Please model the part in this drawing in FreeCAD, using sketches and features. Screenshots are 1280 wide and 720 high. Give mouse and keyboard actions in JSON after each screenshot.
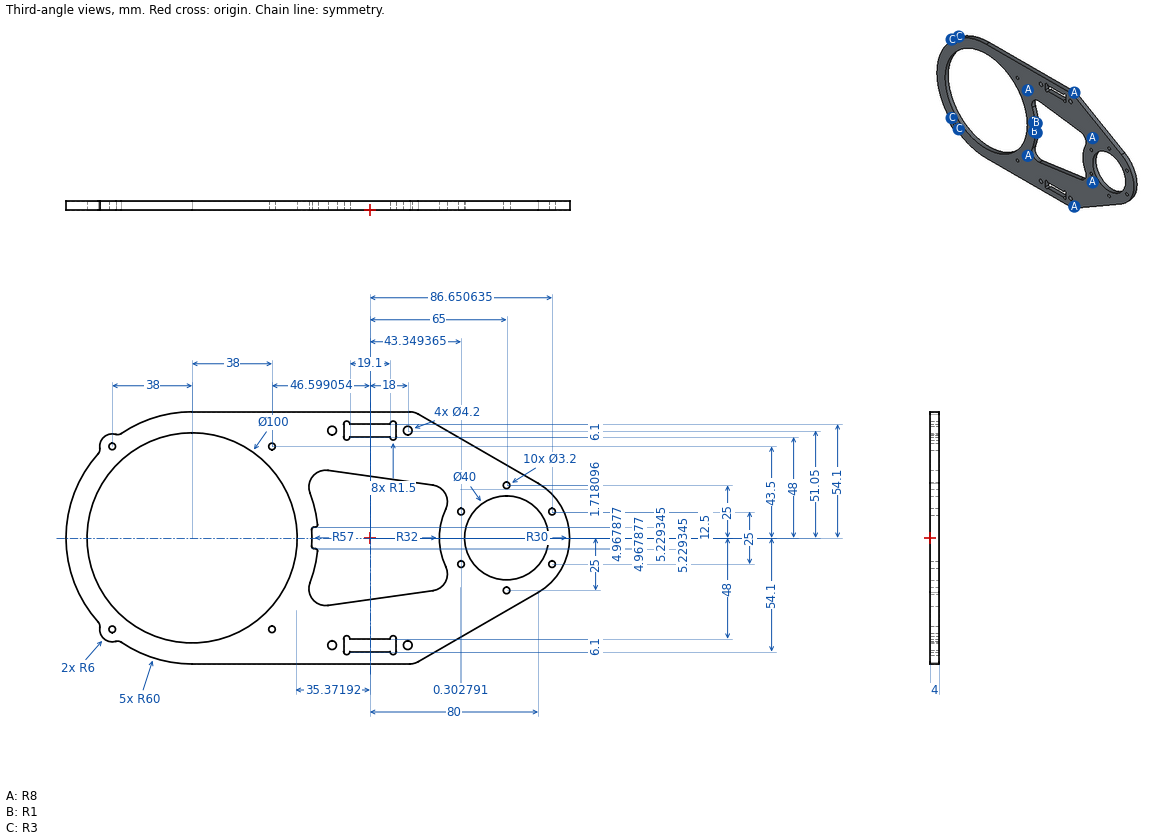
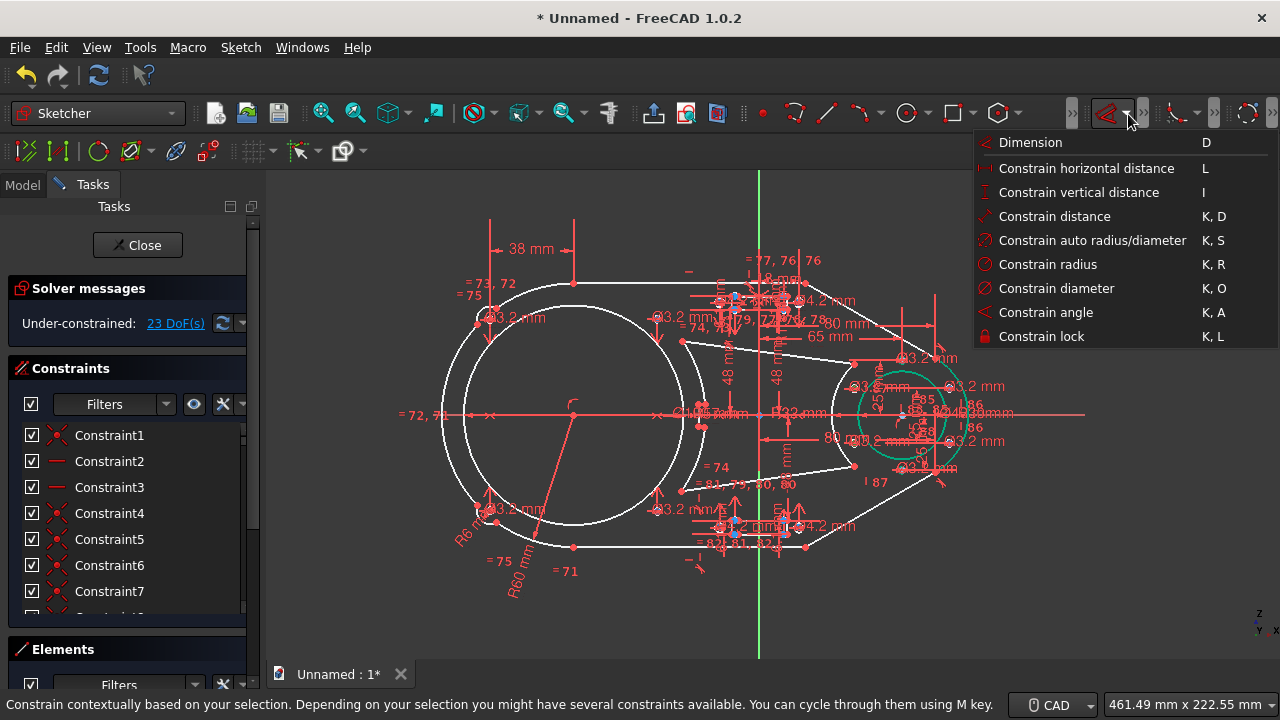
{"action": "left_click", "coordinate": [1126, 192]}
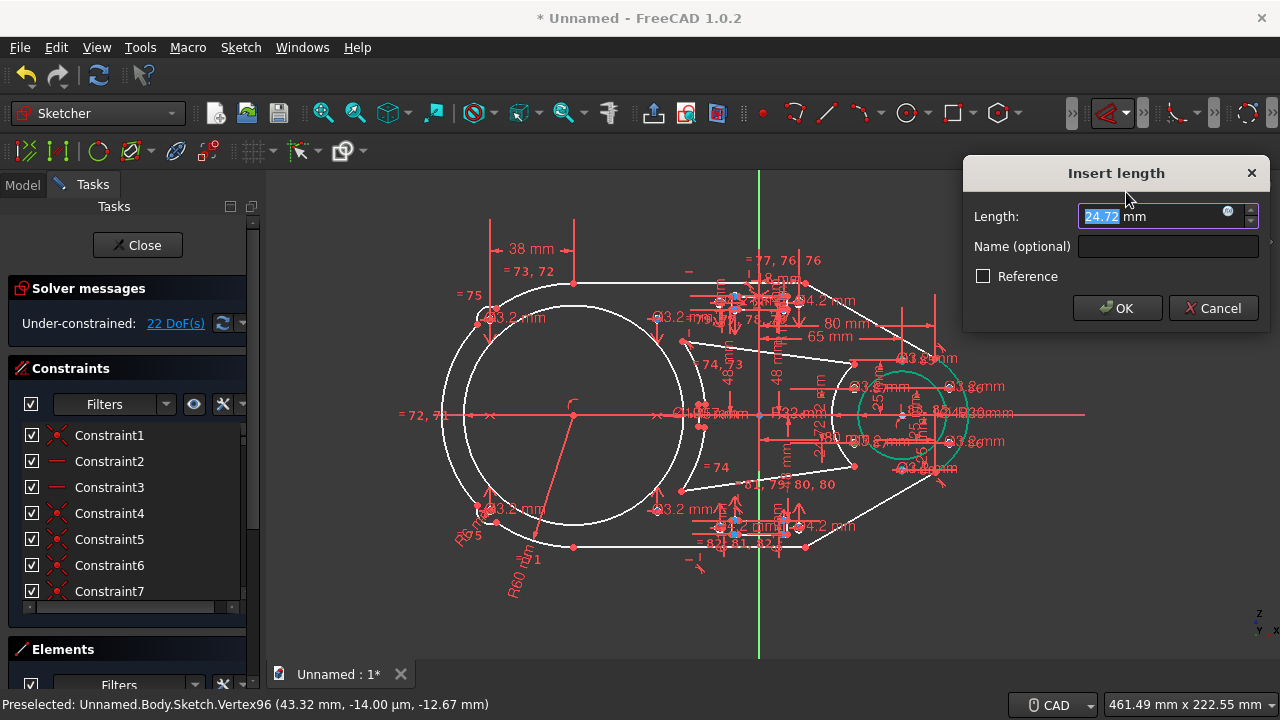
{"action": "type", "text": "25"}
{"action": "key", "text": "Return"}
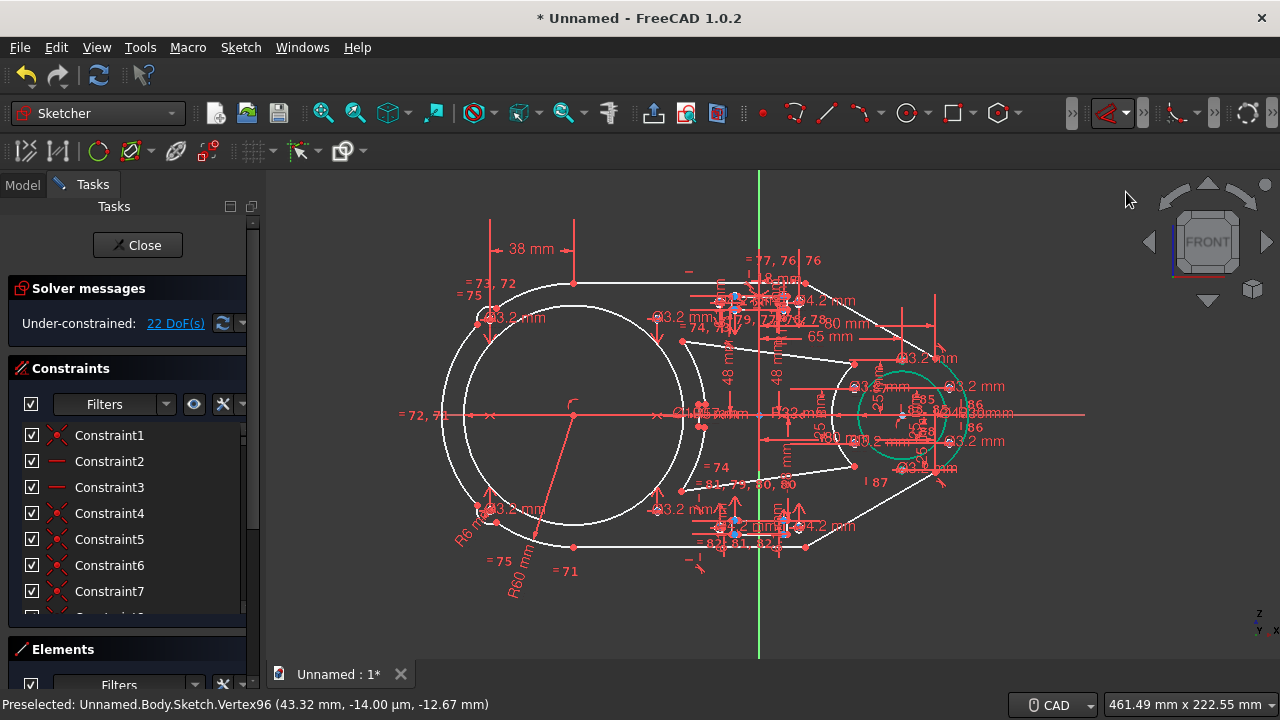
{"action": "left_click", "coordinate": [490, 320]}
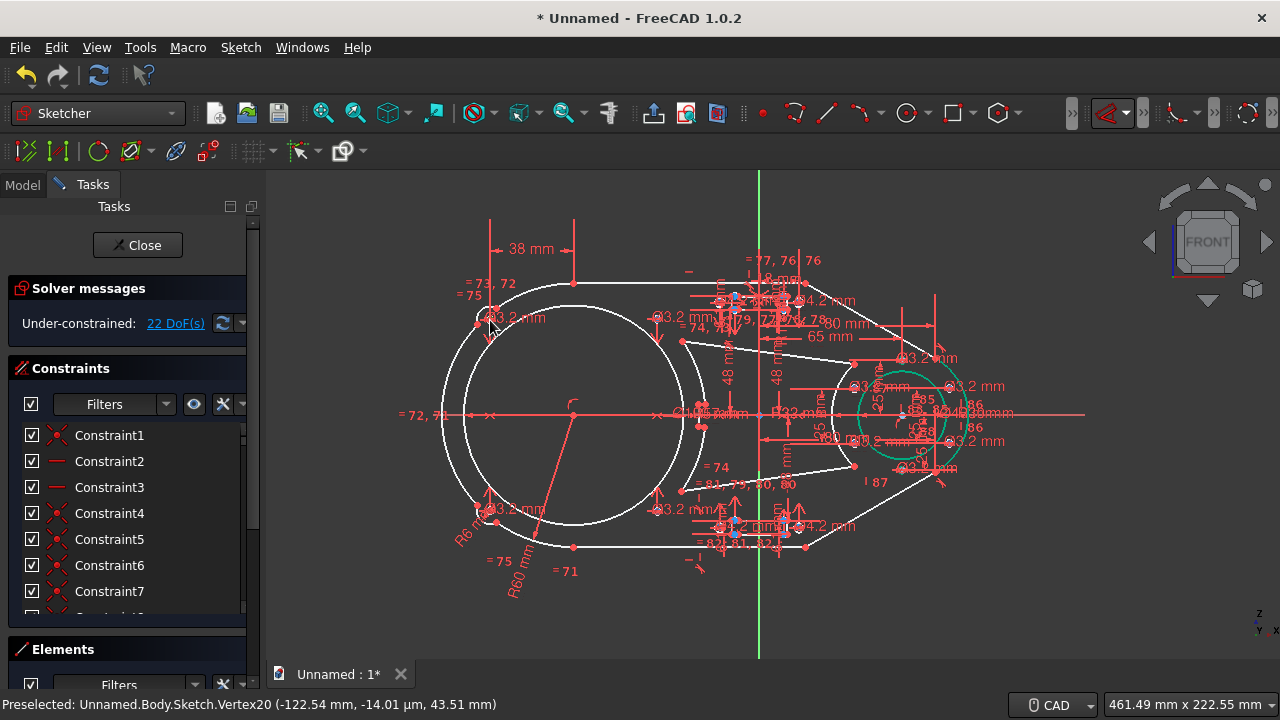
{"action": "left_click", "coordinate": [574, 415]}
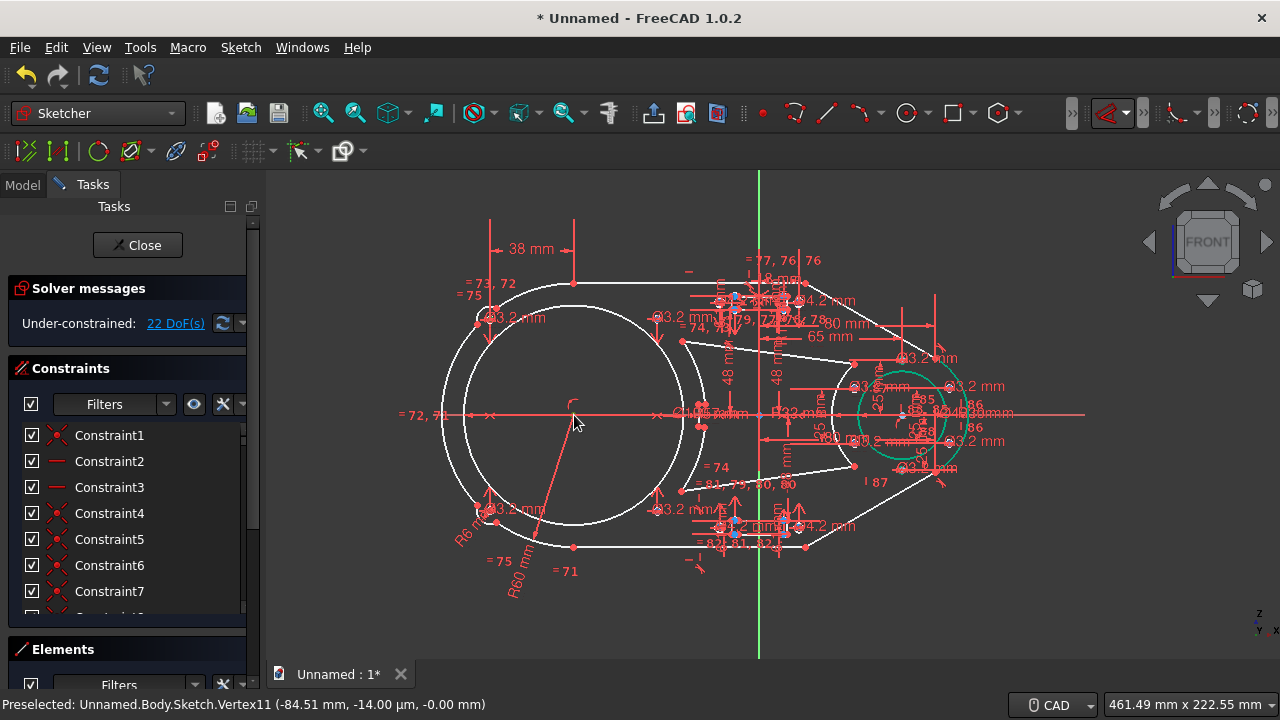
{"action": "left_click", "coordinate": [1128, 114]}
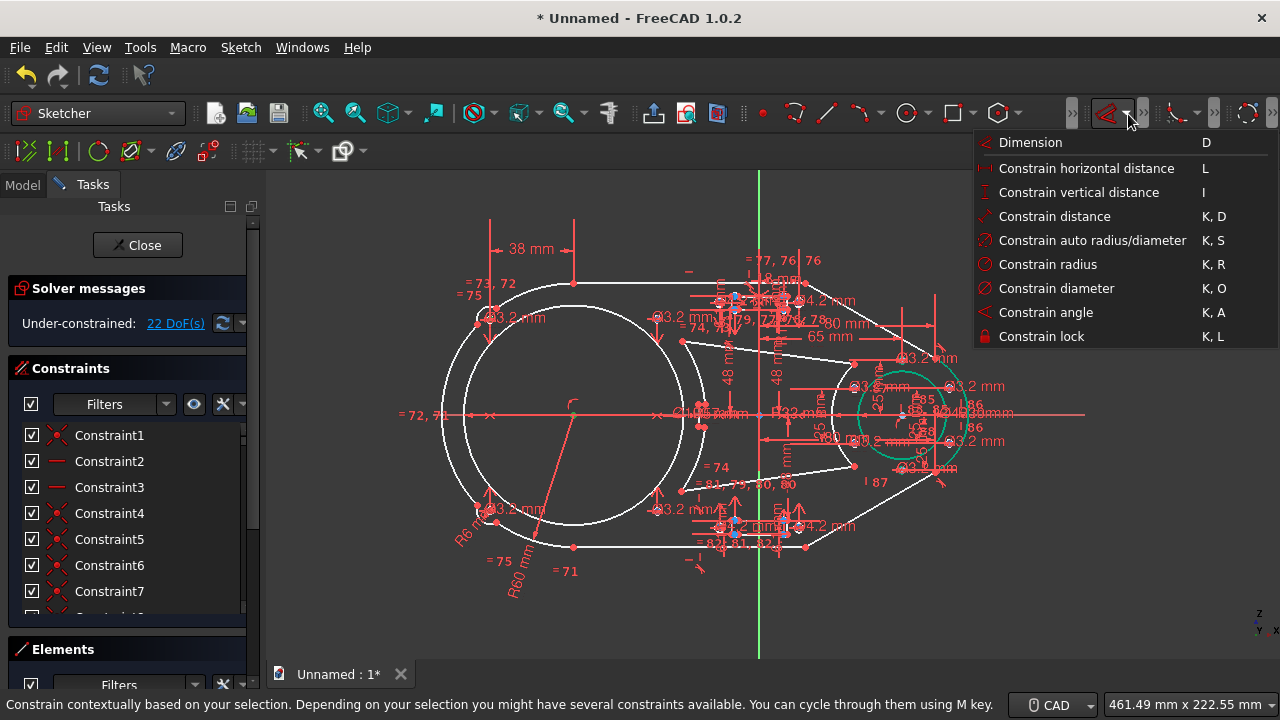
{"action": "left_click", "coordinate": [1126, 168]}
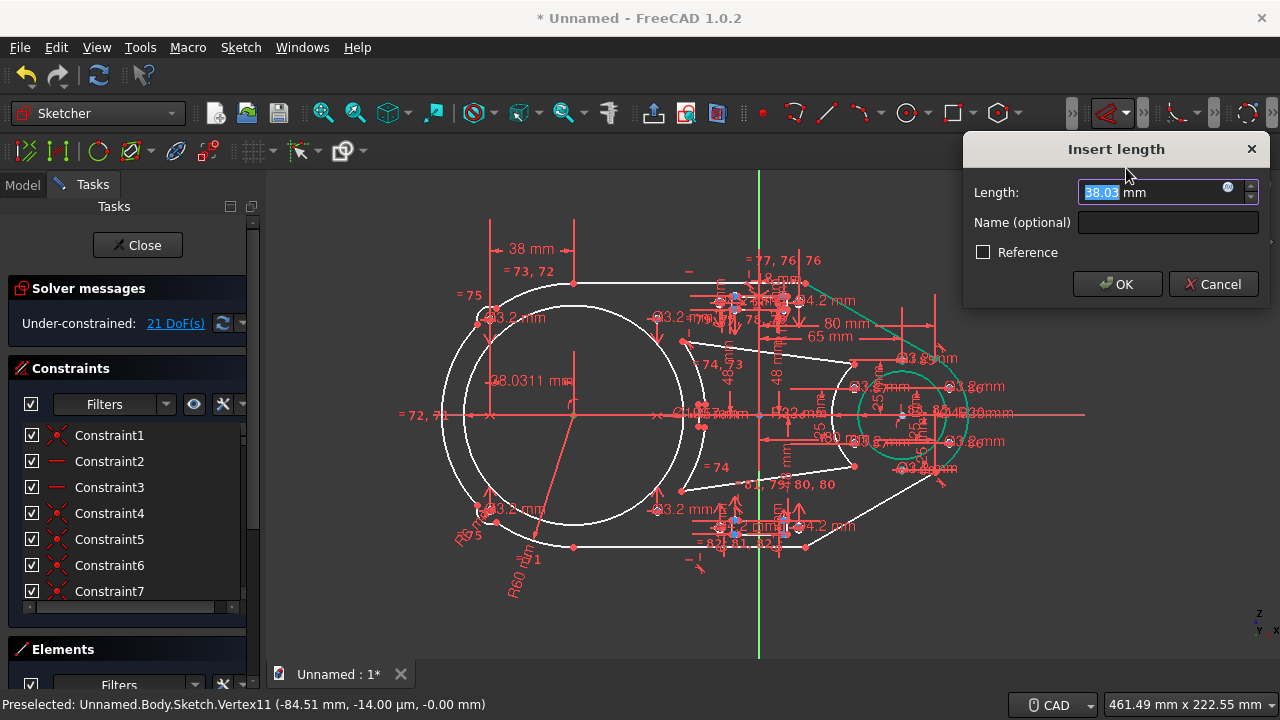
{"action": "type", "text": "38"}
{"action": "key", "text": "Return"}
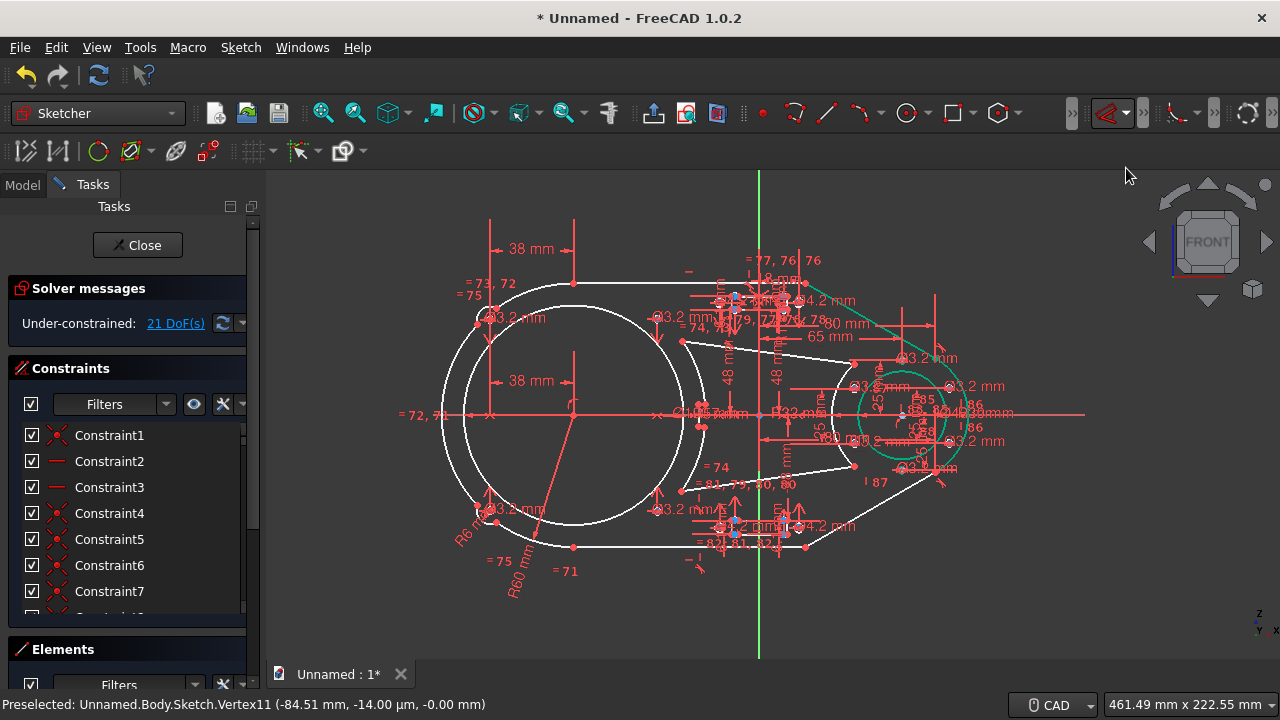
{"action": "left_click", "coordinate": [657, 319]}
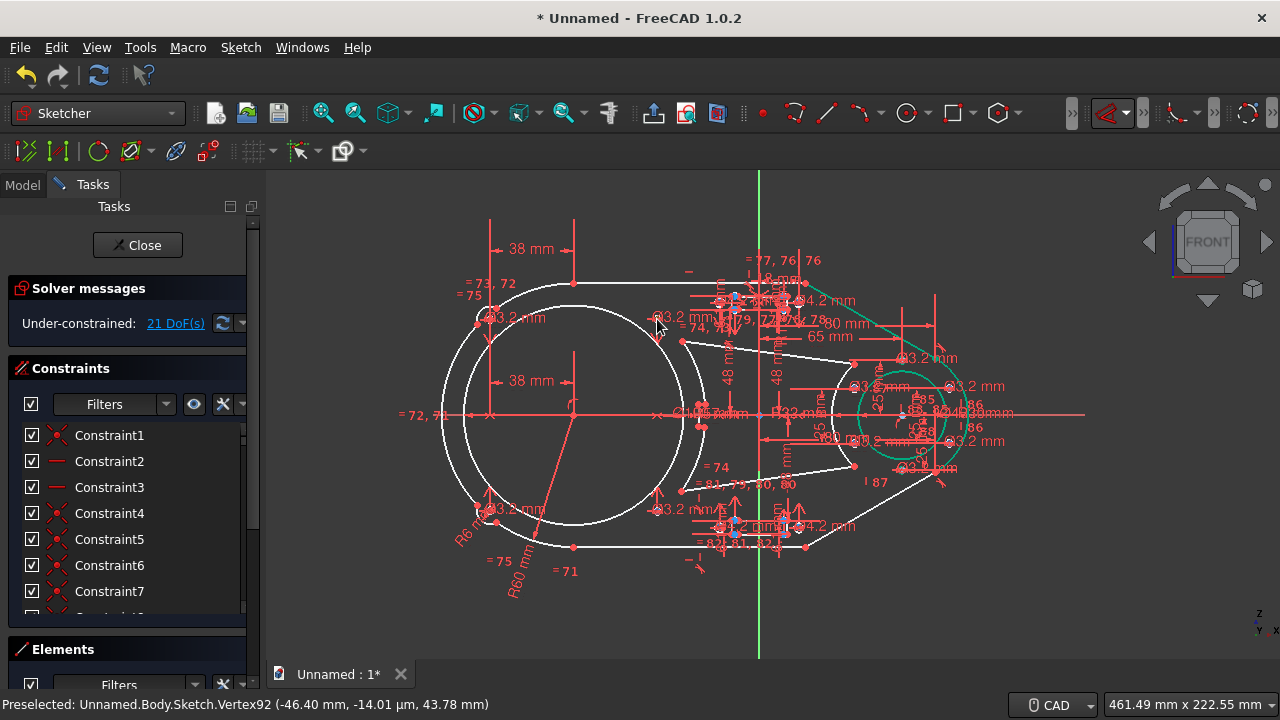
{"action": "left_click", "coordinate": [574, 415]}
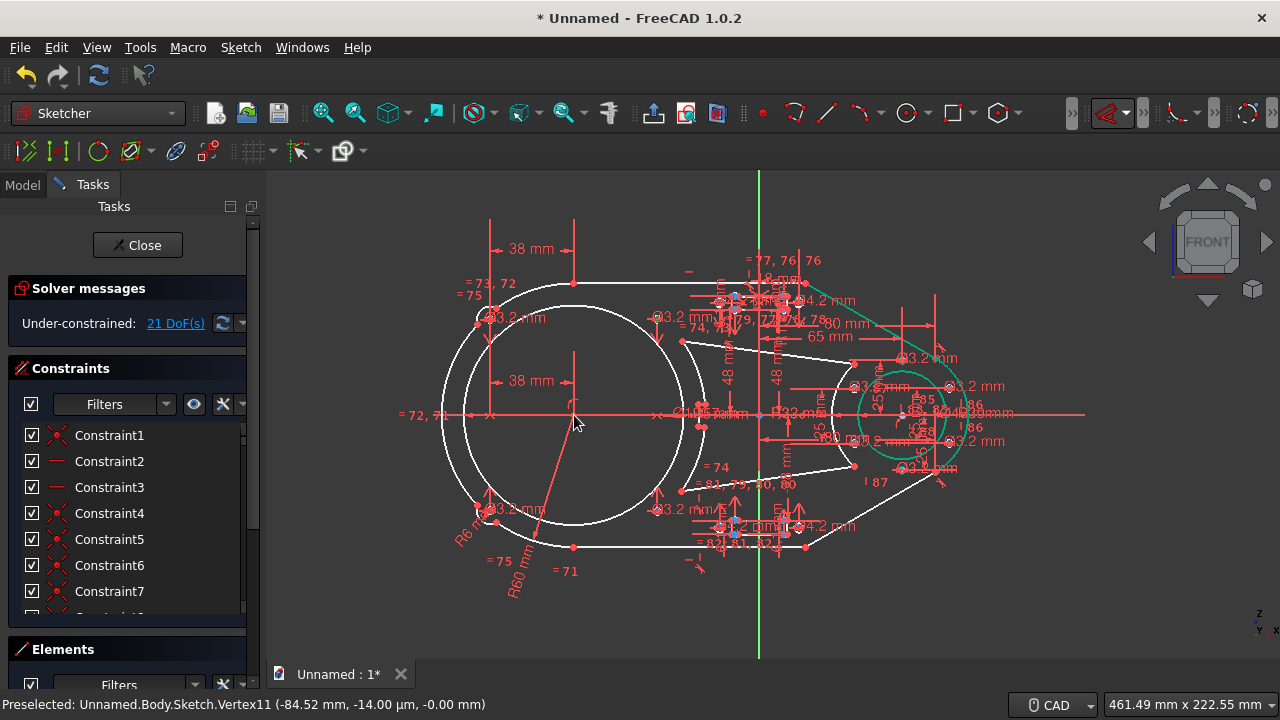
{"action": "key", "text": "l"}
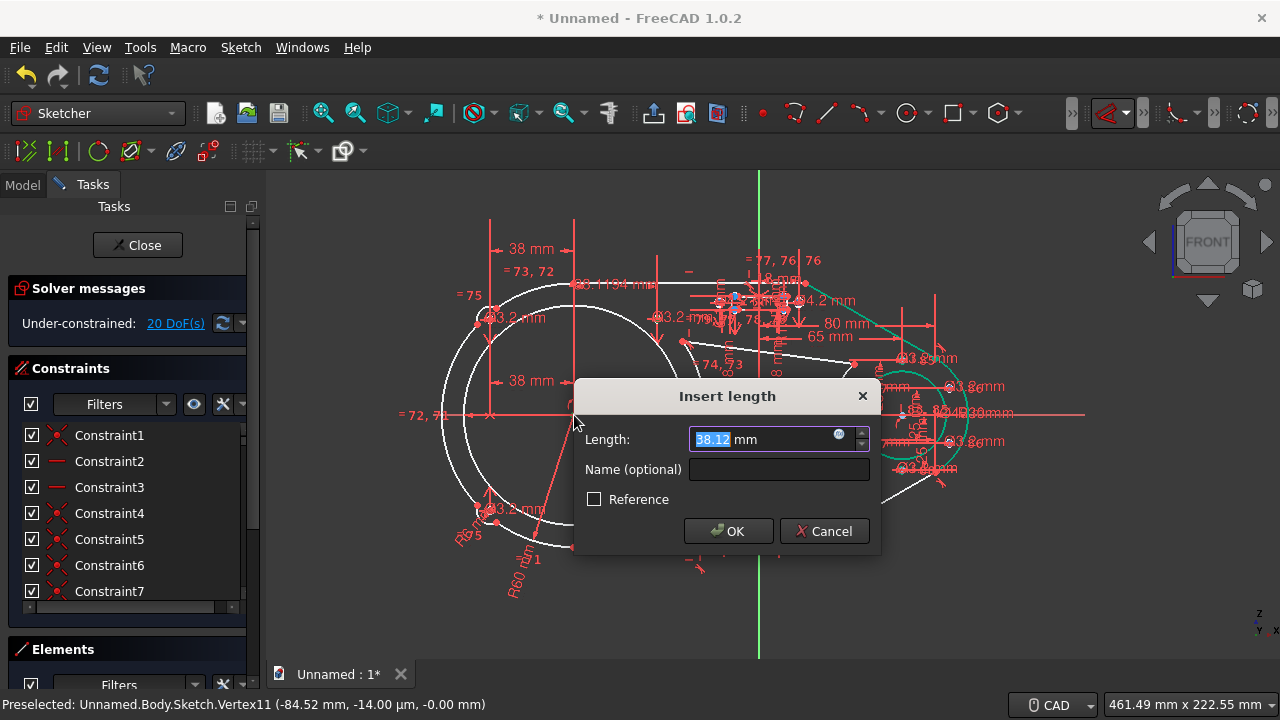
{"action": "type", "text": "38"}
{"action": "key", "text": "Return"}